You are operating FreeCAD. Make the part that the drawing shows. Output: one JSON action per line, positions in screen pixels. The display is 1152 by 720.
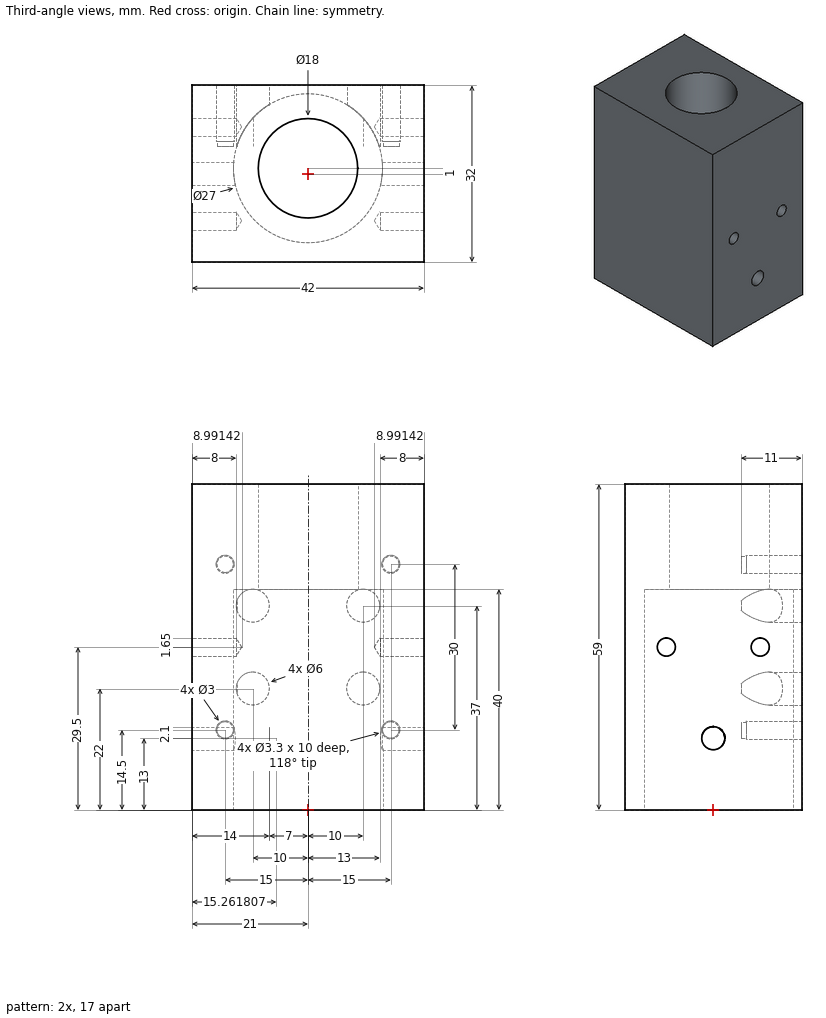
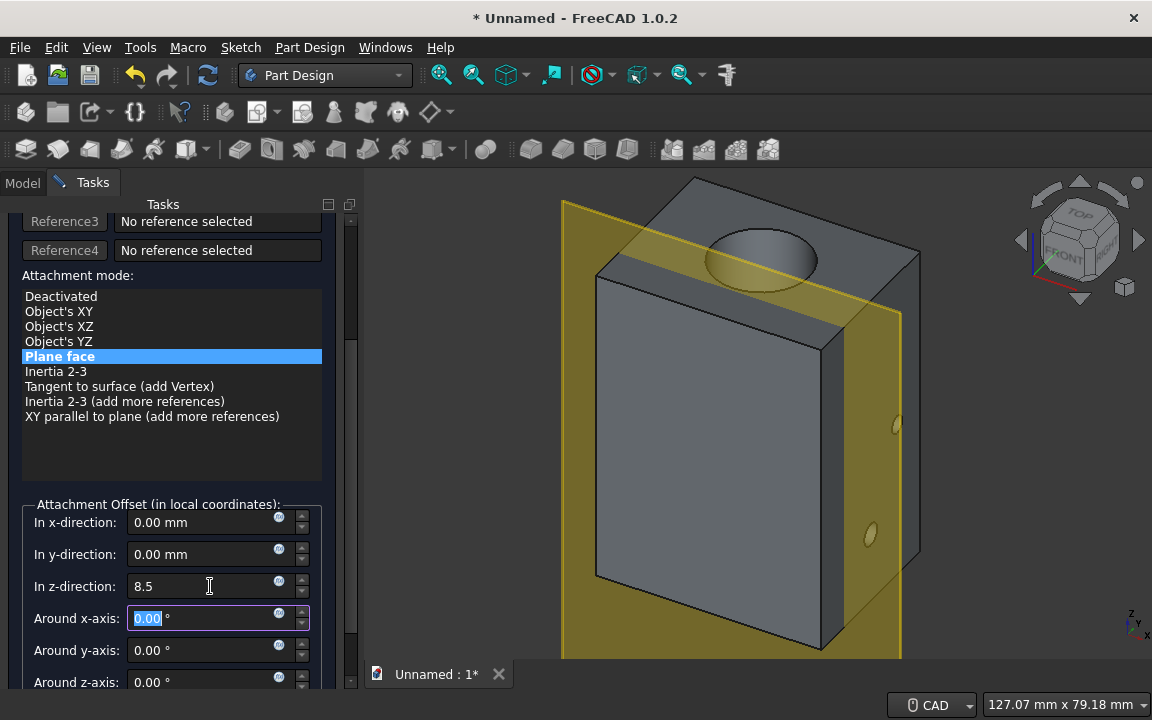
{"action": "scroll", "coordinate": [351, 451], "scroll_direction": "up", "scroll_amount": 4}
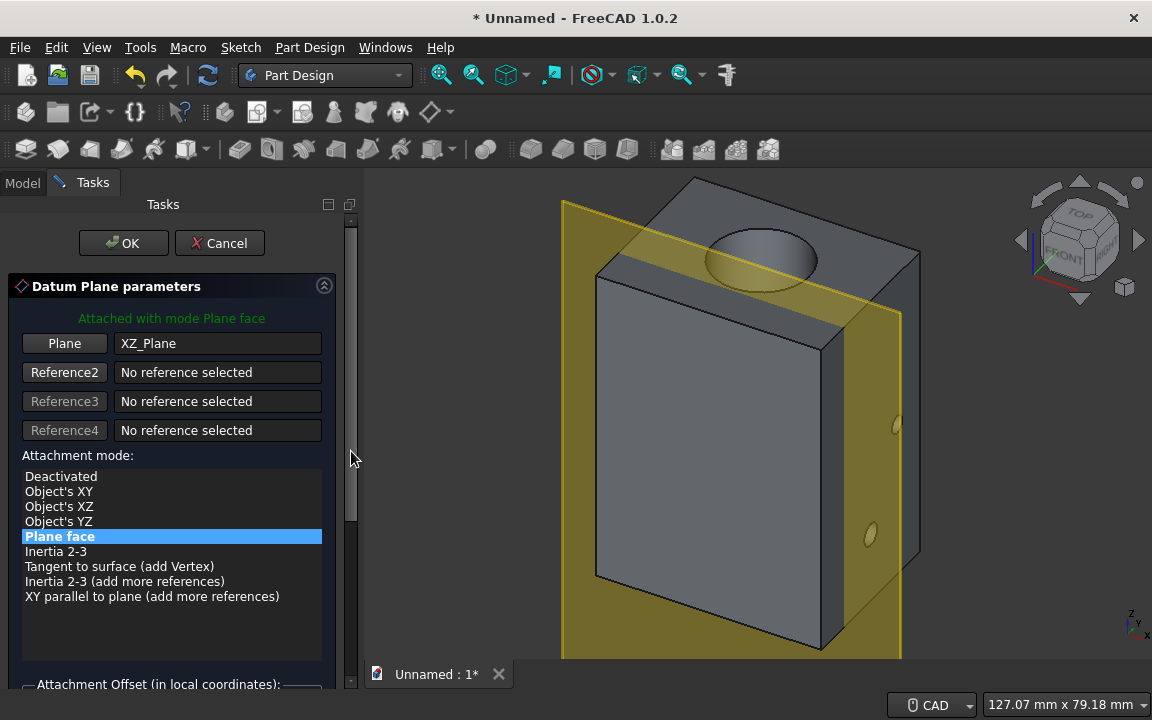
{"action": "left_click", "coordinate": [124, 243]}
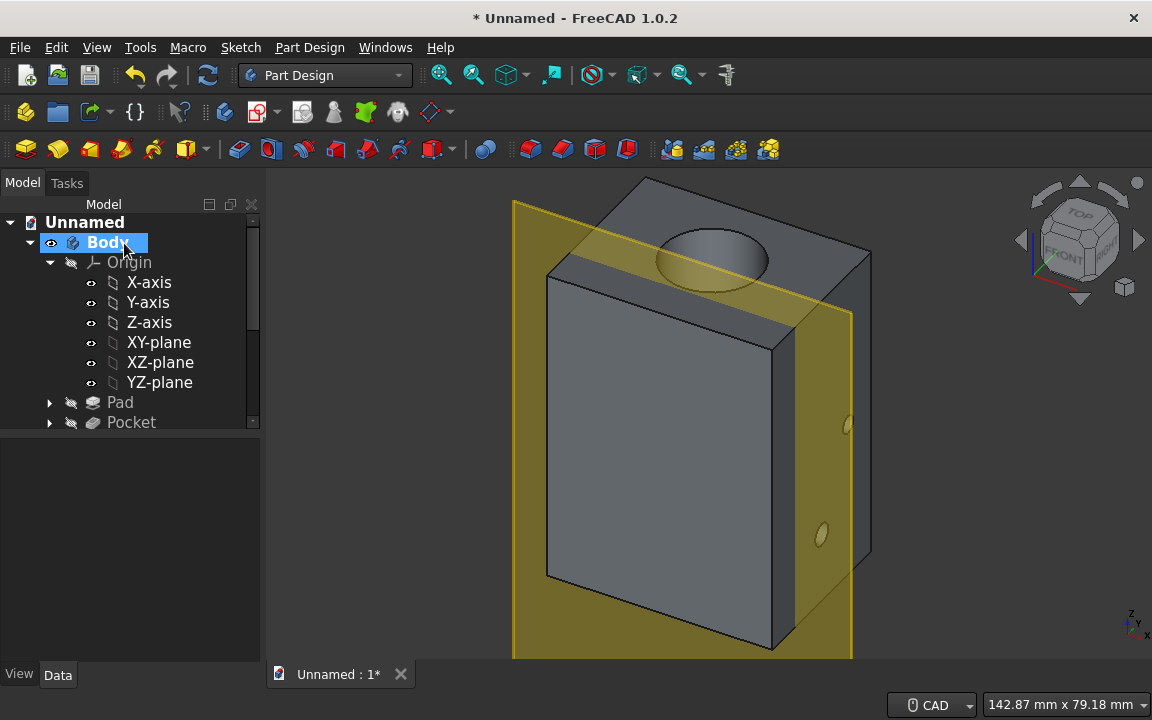
{"action": "scroll", "coordinate": [100, 318], "scroll_direction": "down", "scroll_amount": 3}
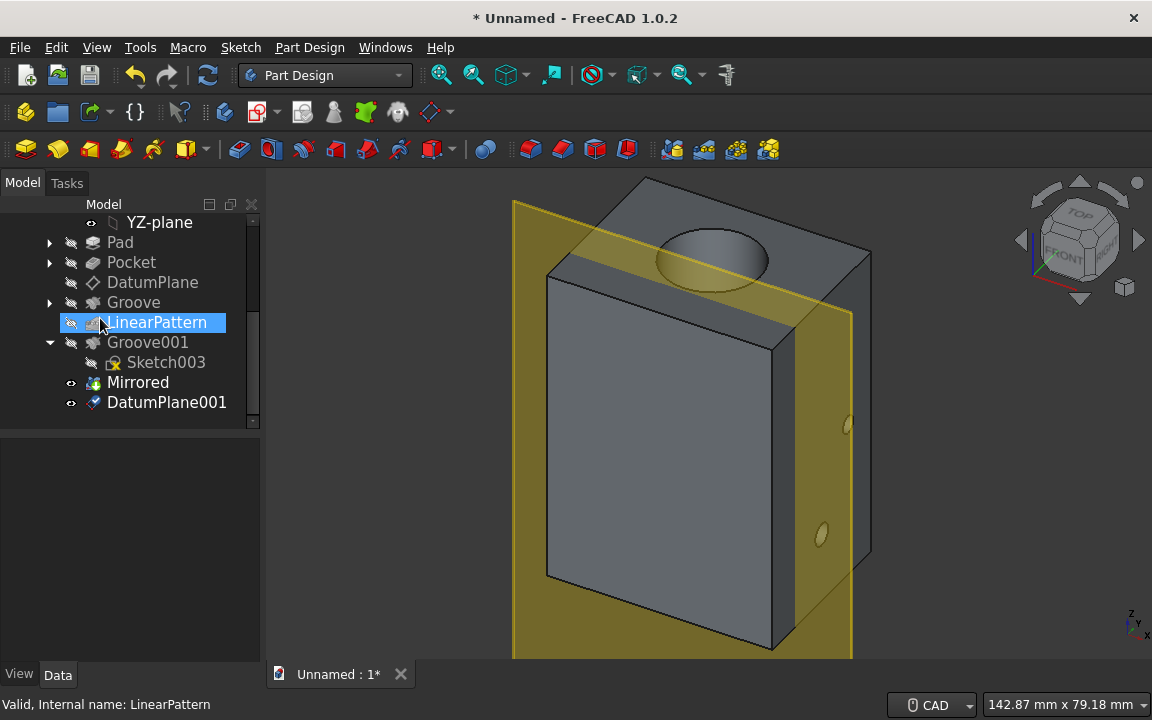
{"action": "left_click", "coordinate": [116, 403]}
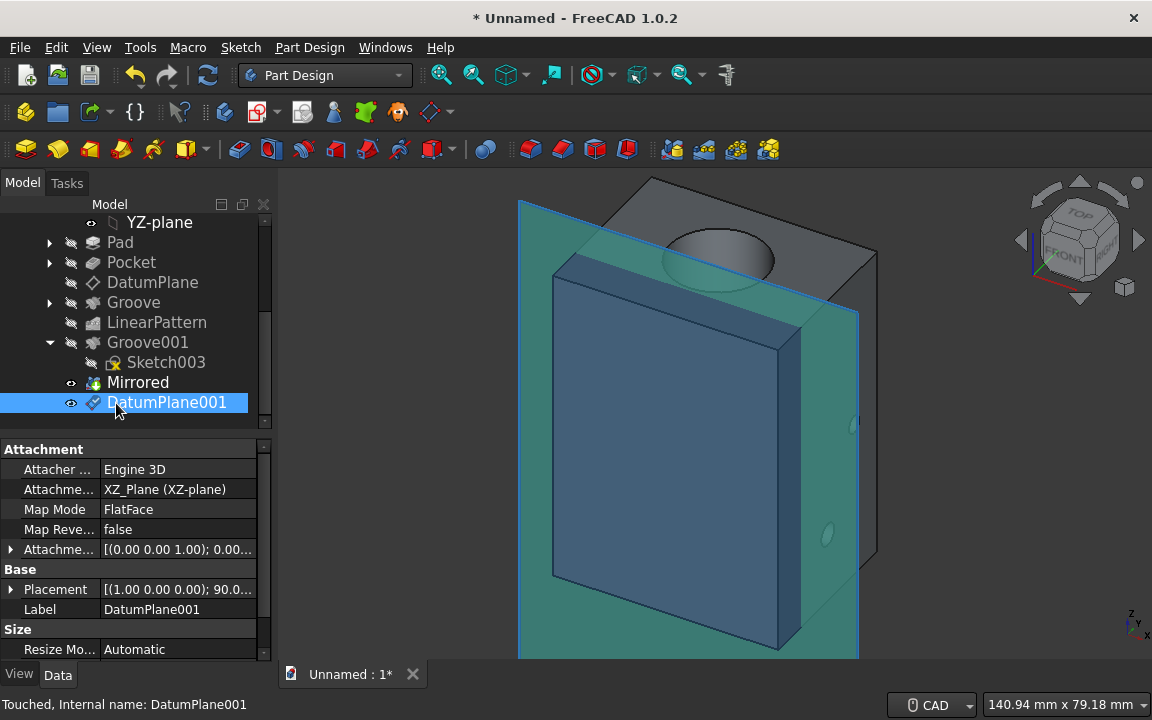
{"action": "left_click", "coordinate": [258, 112]}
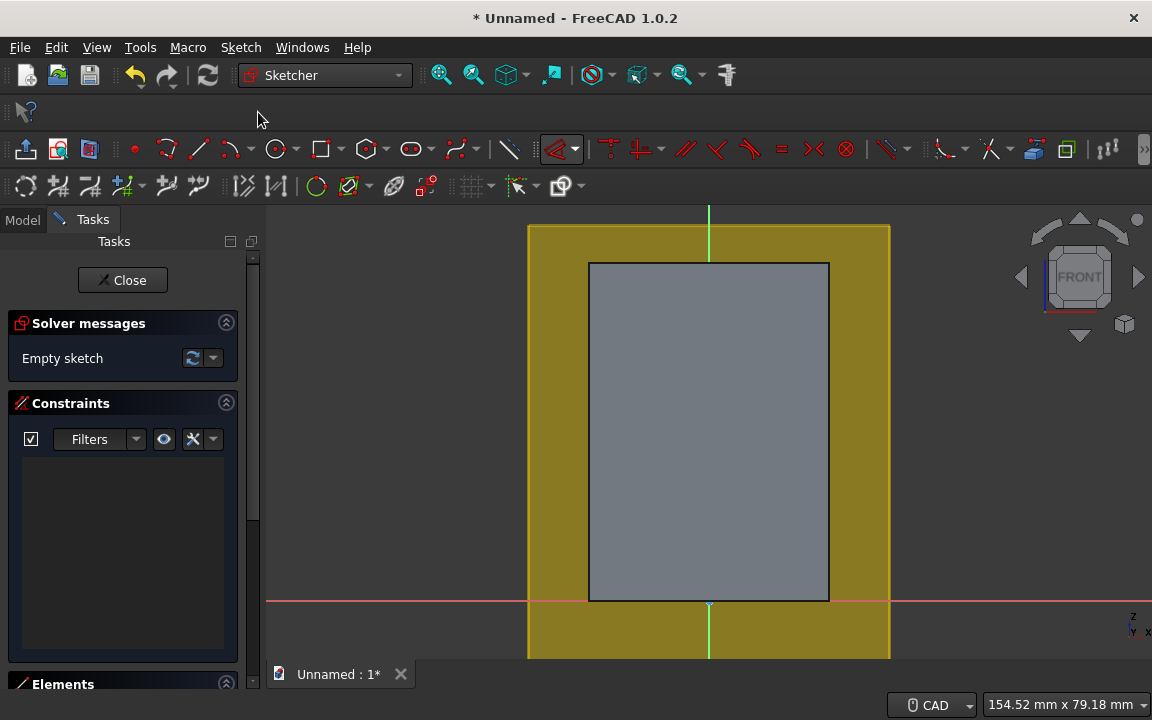
{"action": "left_click", "coordinate": [90, 150]}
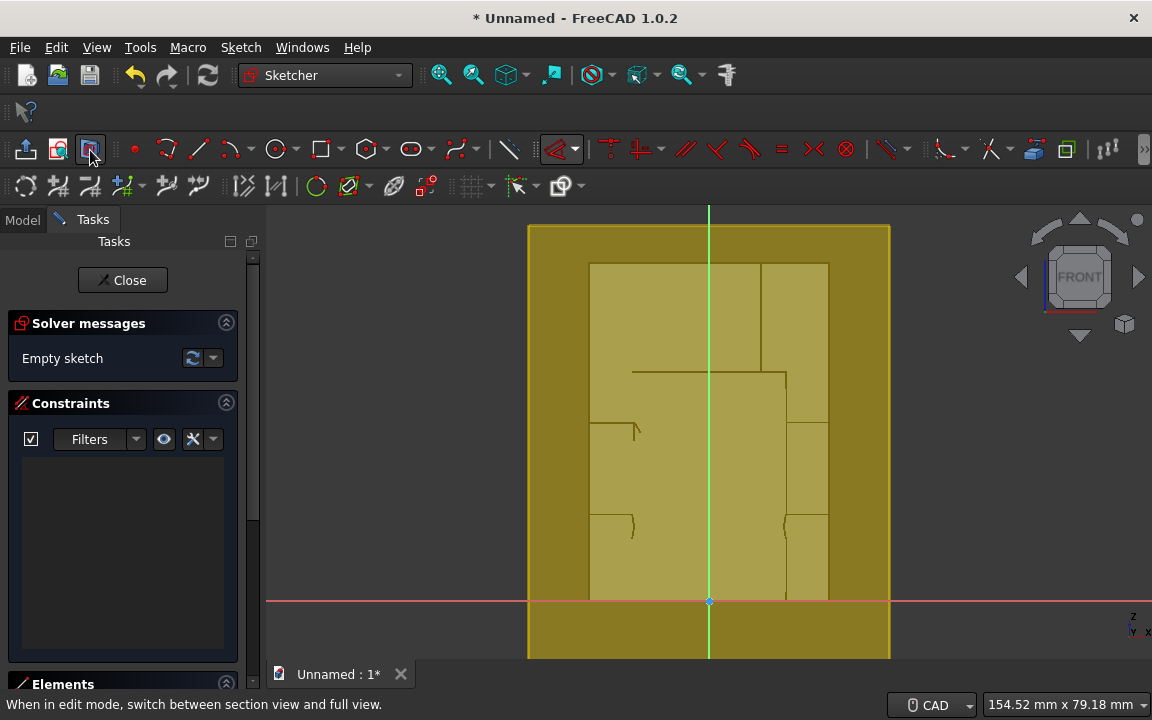
{"action": "scroll", "coordinate": [987, 631], "scroll_direction": "up", "scroll_amount": 2}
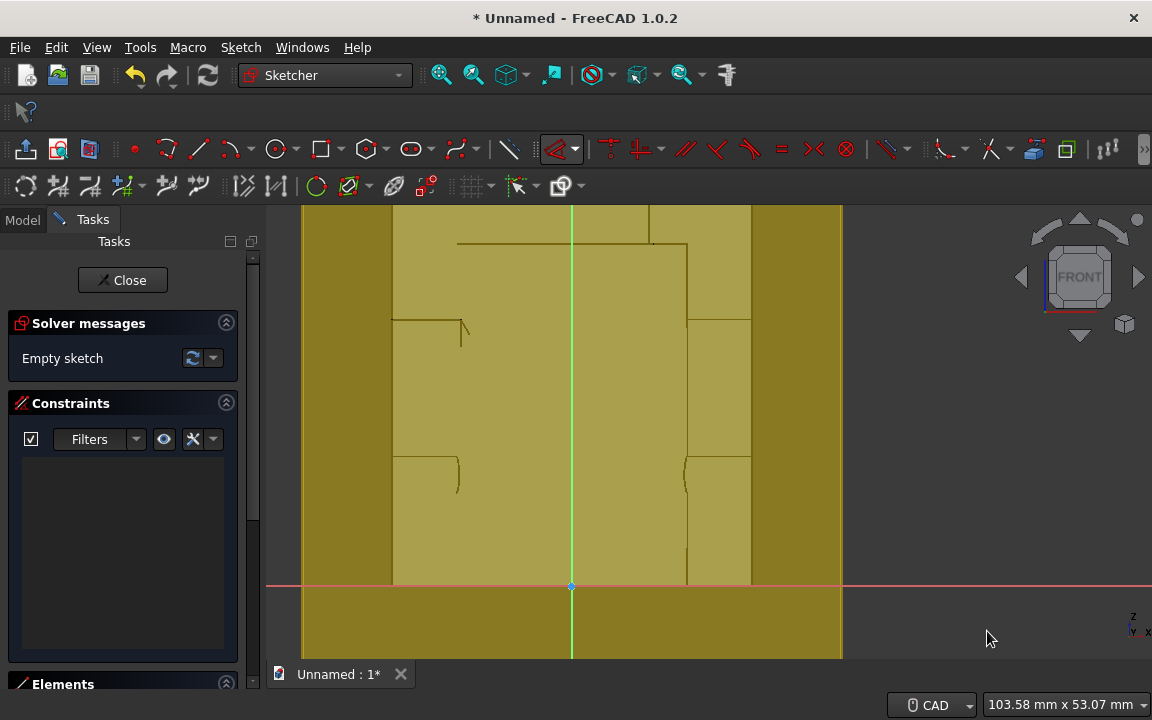
{"action": "key", "text": "g m"}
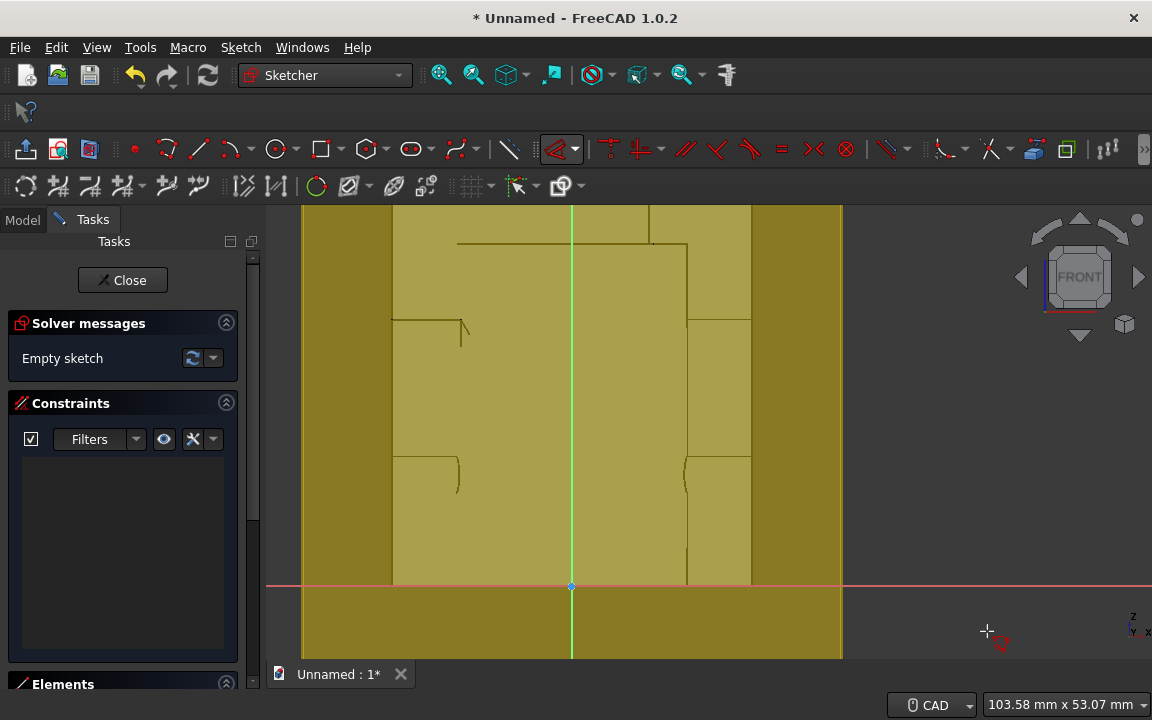
{"action": "left_click", "coordinate": [675, 334]}
{"action": "left_click", "coordinate": [683, 320]}
{"action": "left_click", "coordinate": [752, 320]}
{"action": "left_click", "coordinate": [752, 334]}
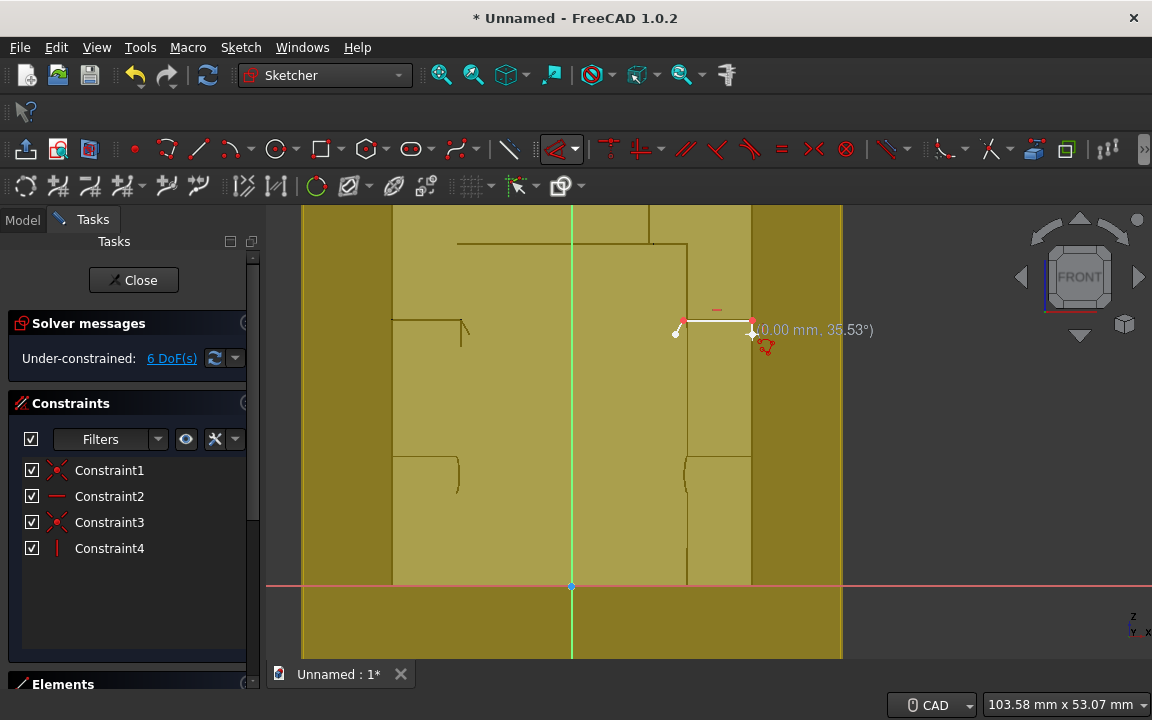
{"action": "scroll", "coordinate": [675, 334], "scroll_direction": "up", "scroll_amount": 4}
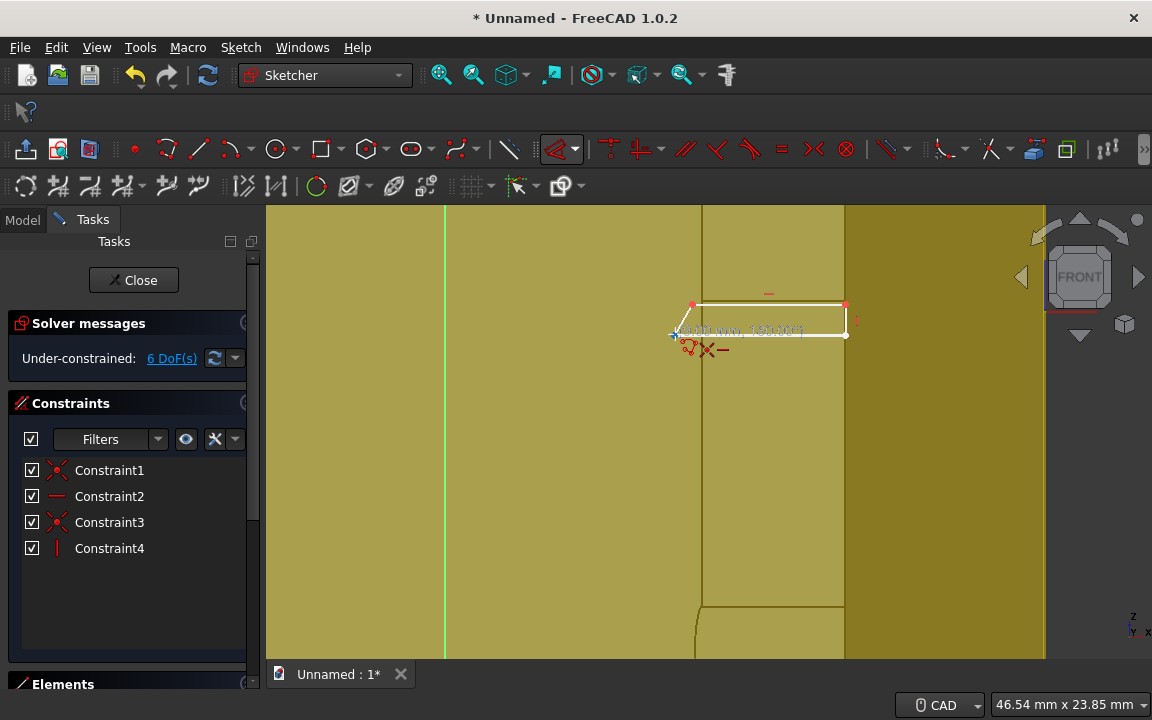
{"action": "left_click", "coordinate": [674, 336]}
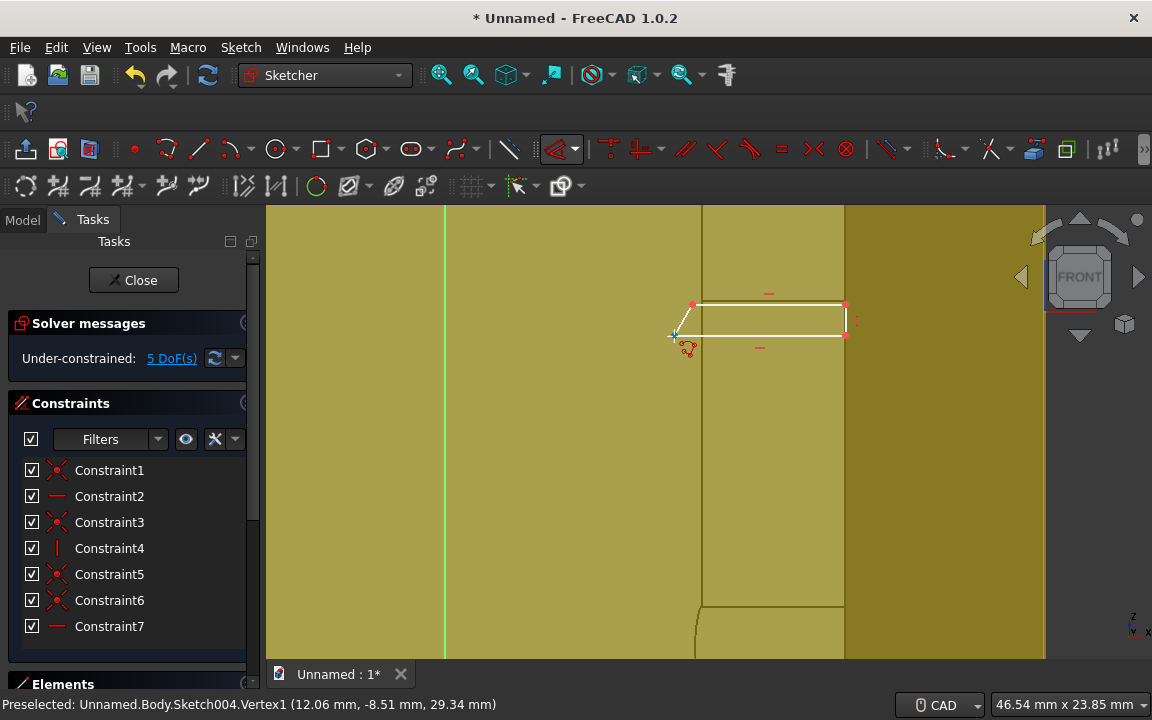
{"action": "key", "text": "g l"}